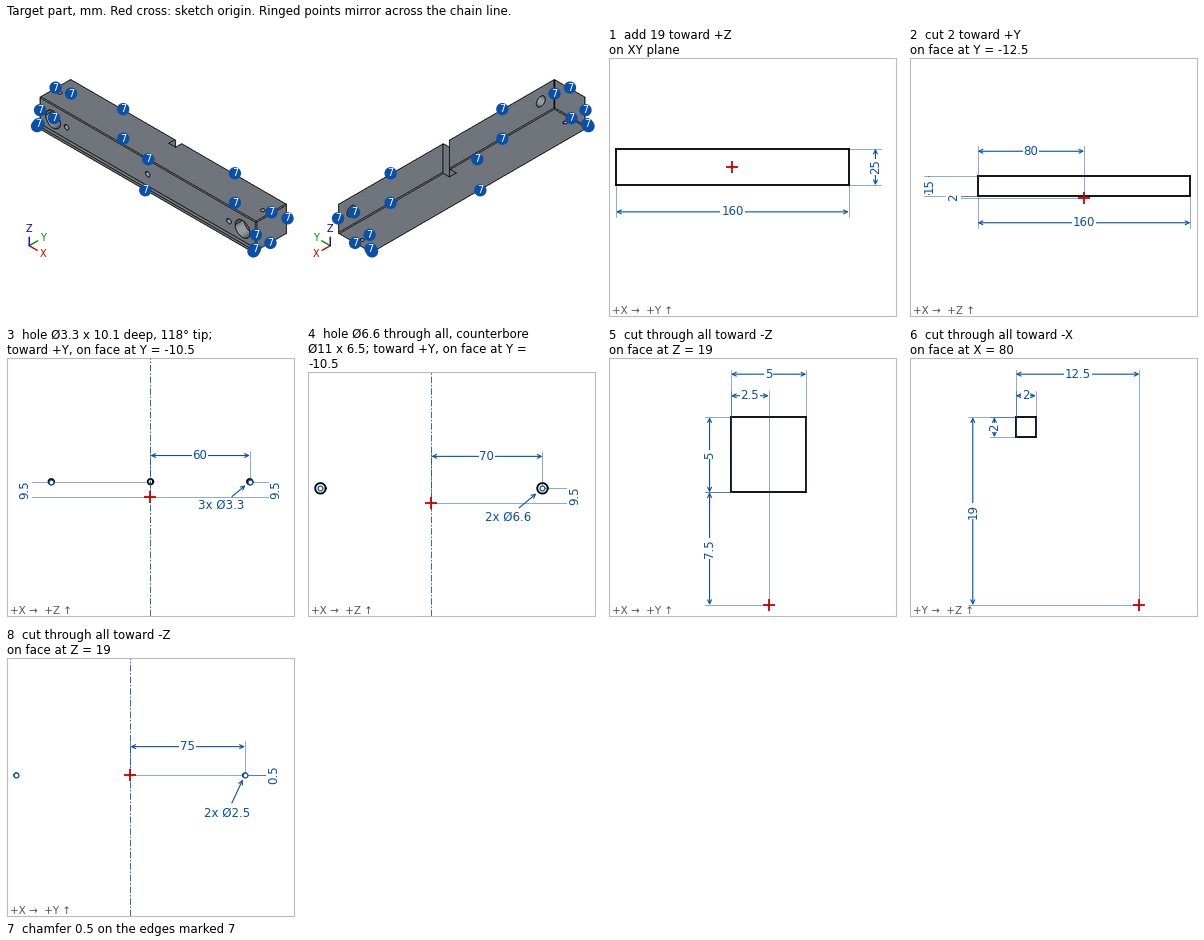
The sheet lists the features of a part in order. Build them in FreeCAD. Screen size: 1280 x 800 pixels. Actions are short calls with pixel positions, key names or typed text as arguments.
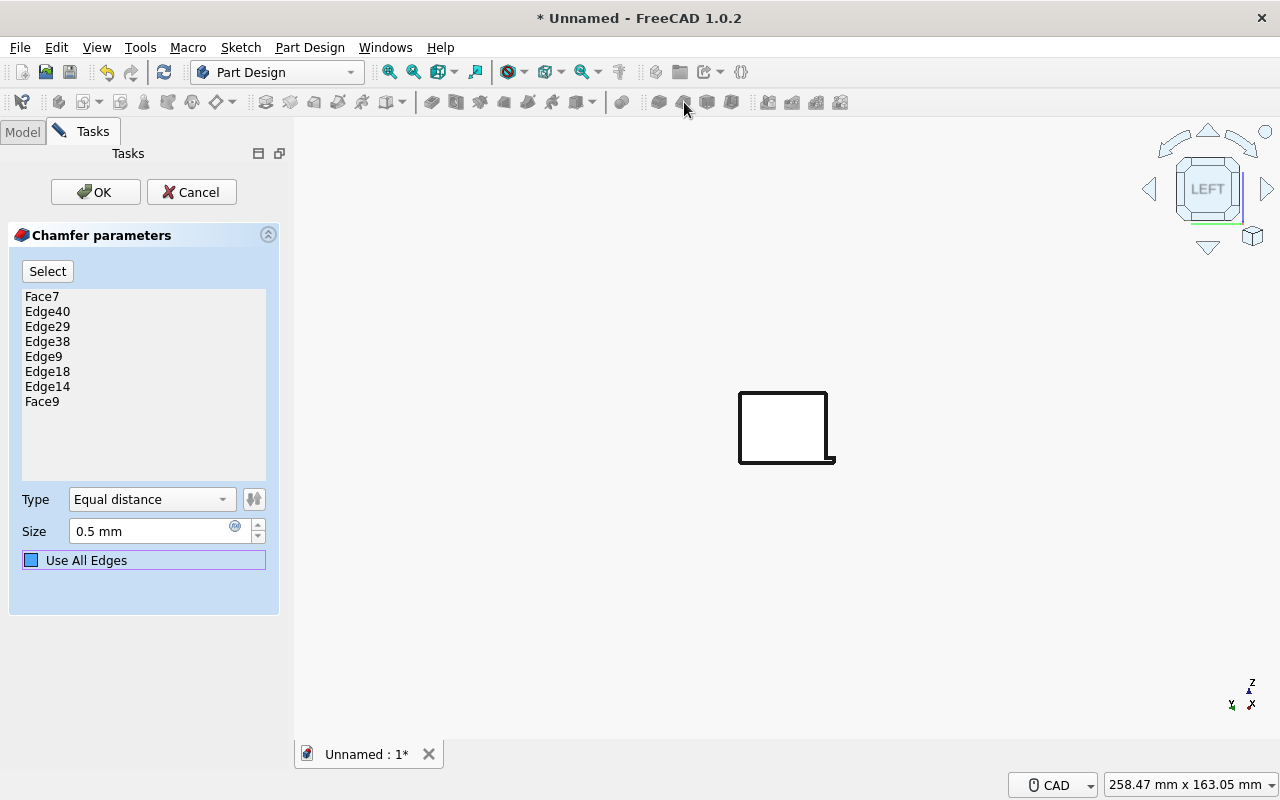
click(96, 192)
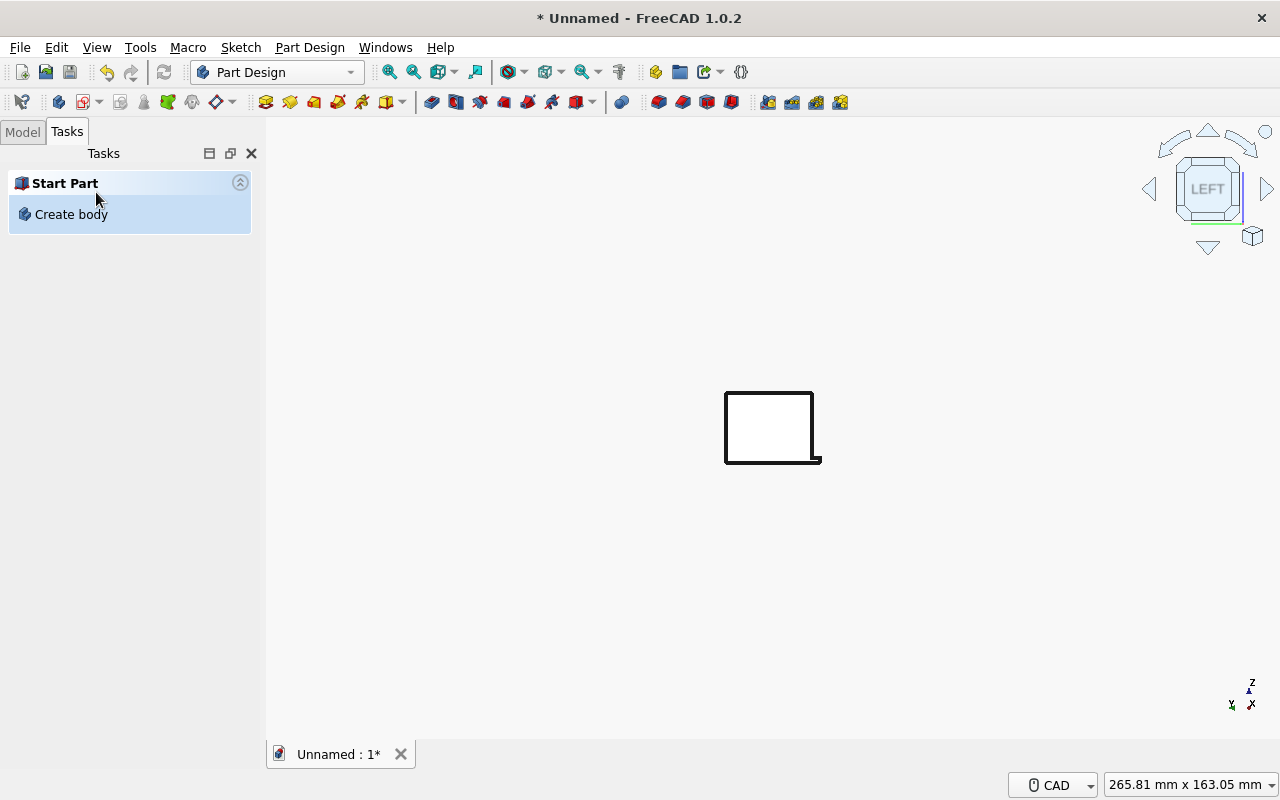
click(390, 72)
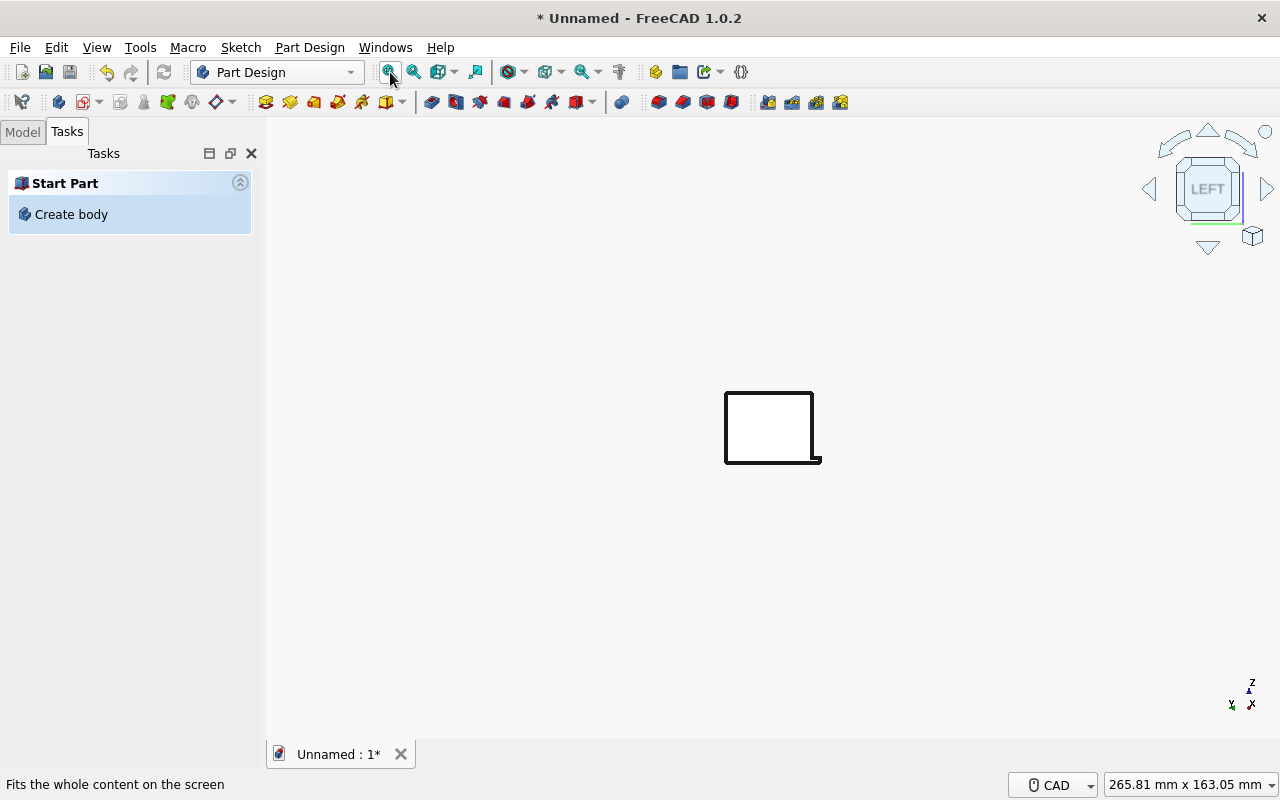
key(0)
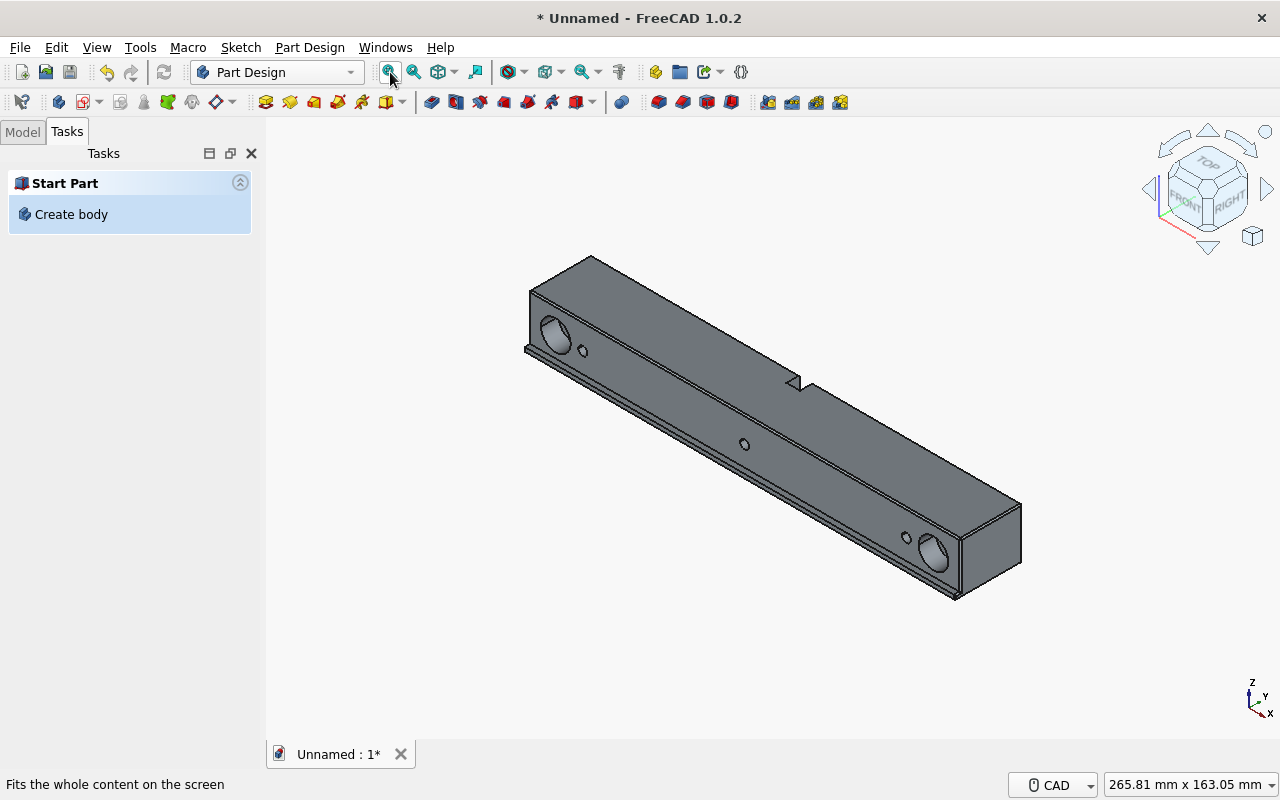
click(960, 502)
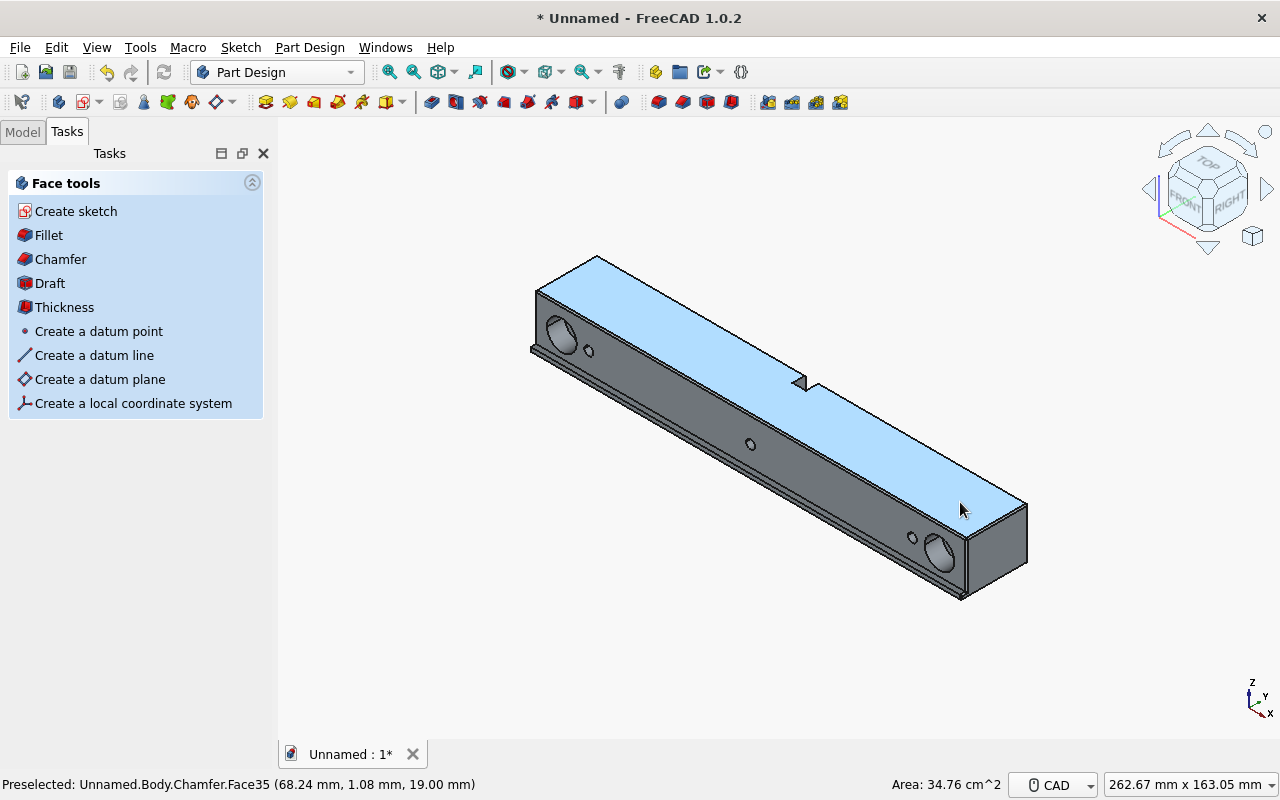
click(84, 102)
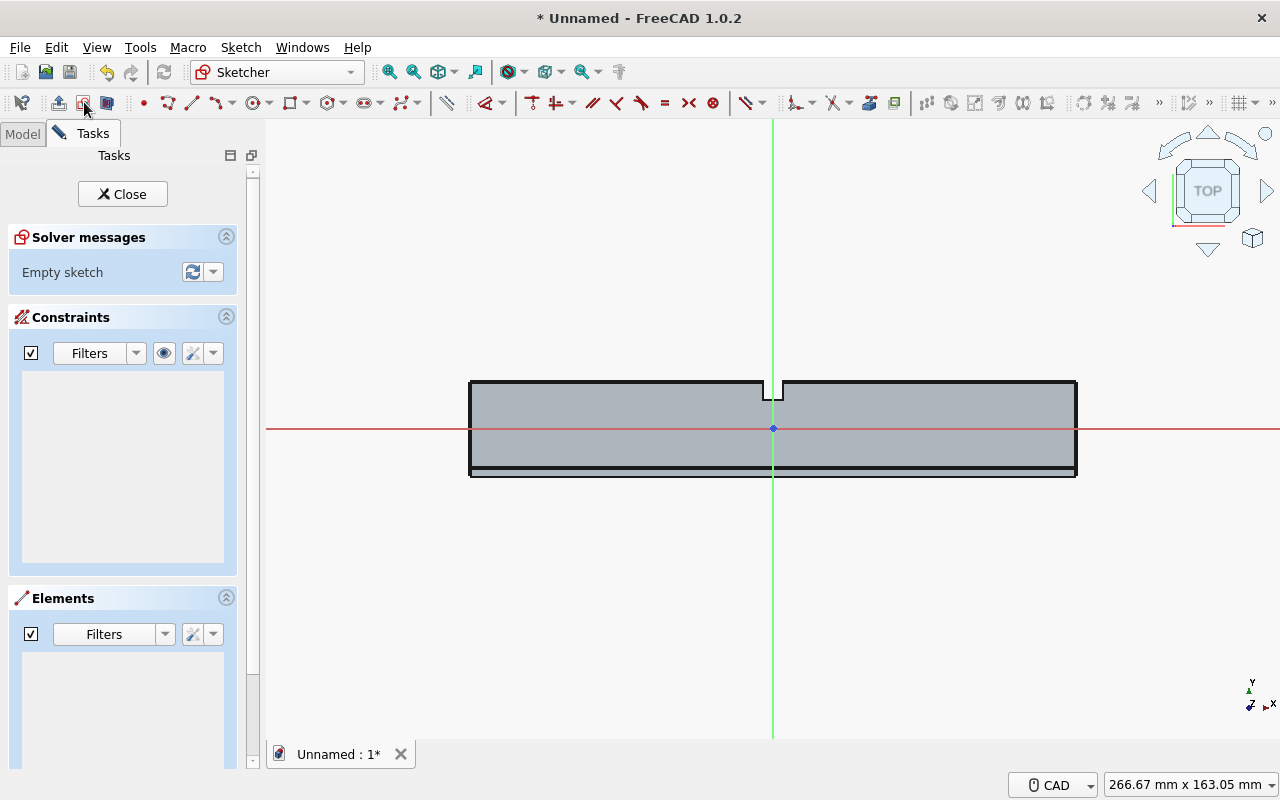
click(254, 104)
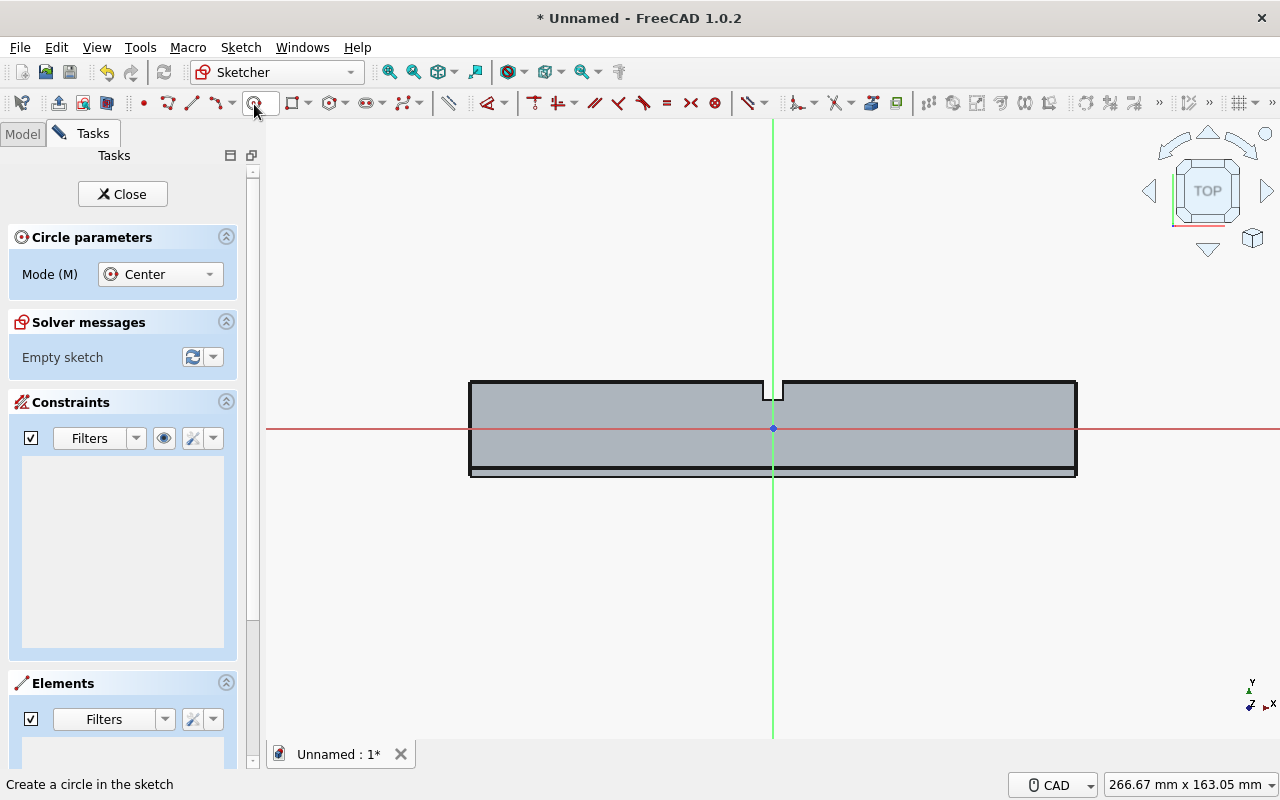
scroll(1058, 431, up, 11)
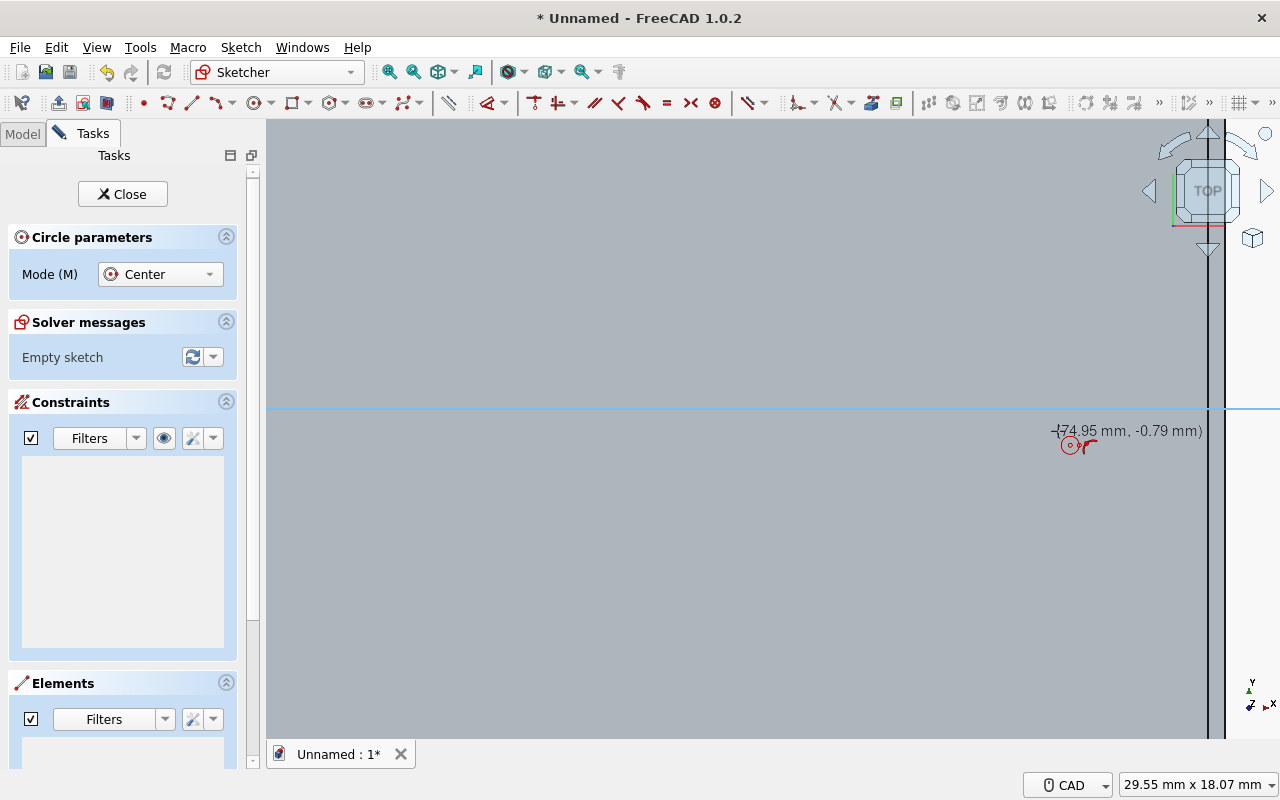
click(1053, 426)
click(1084, 456)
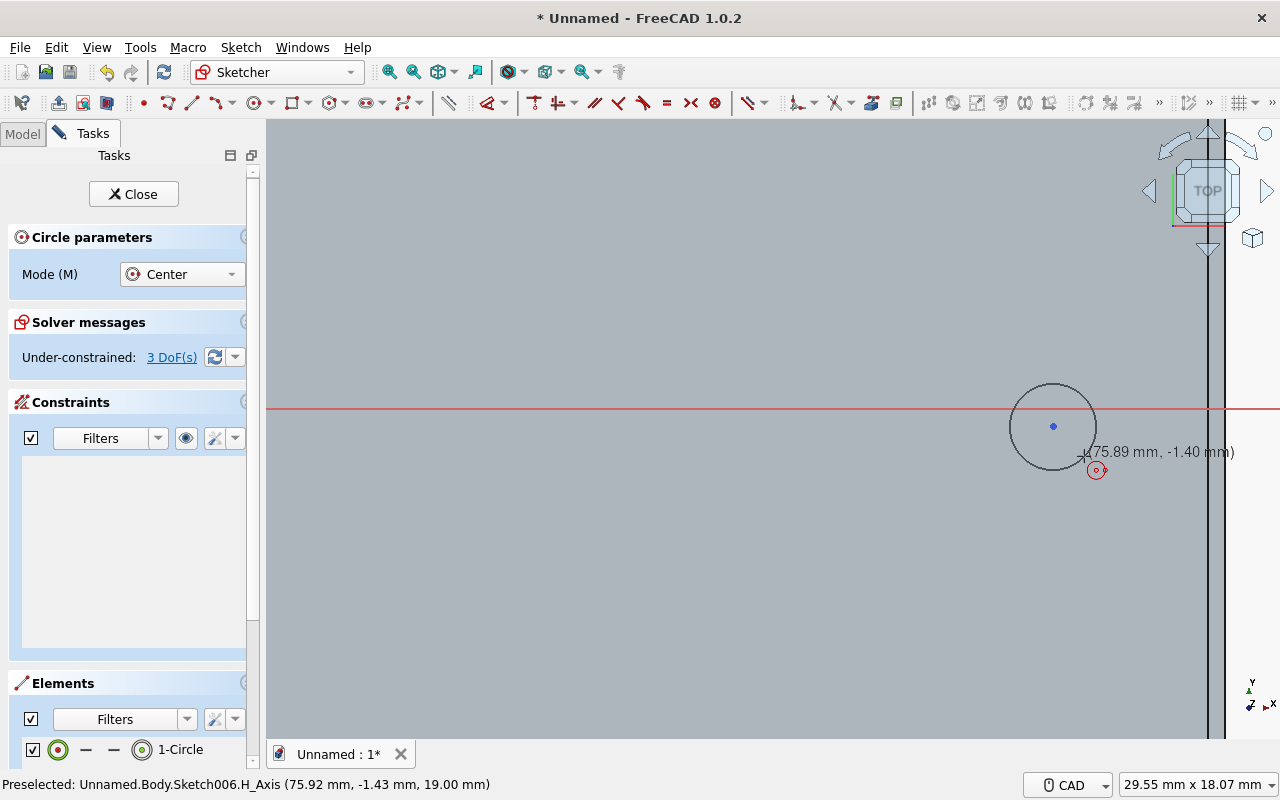
scroll(982, 429, down, 11)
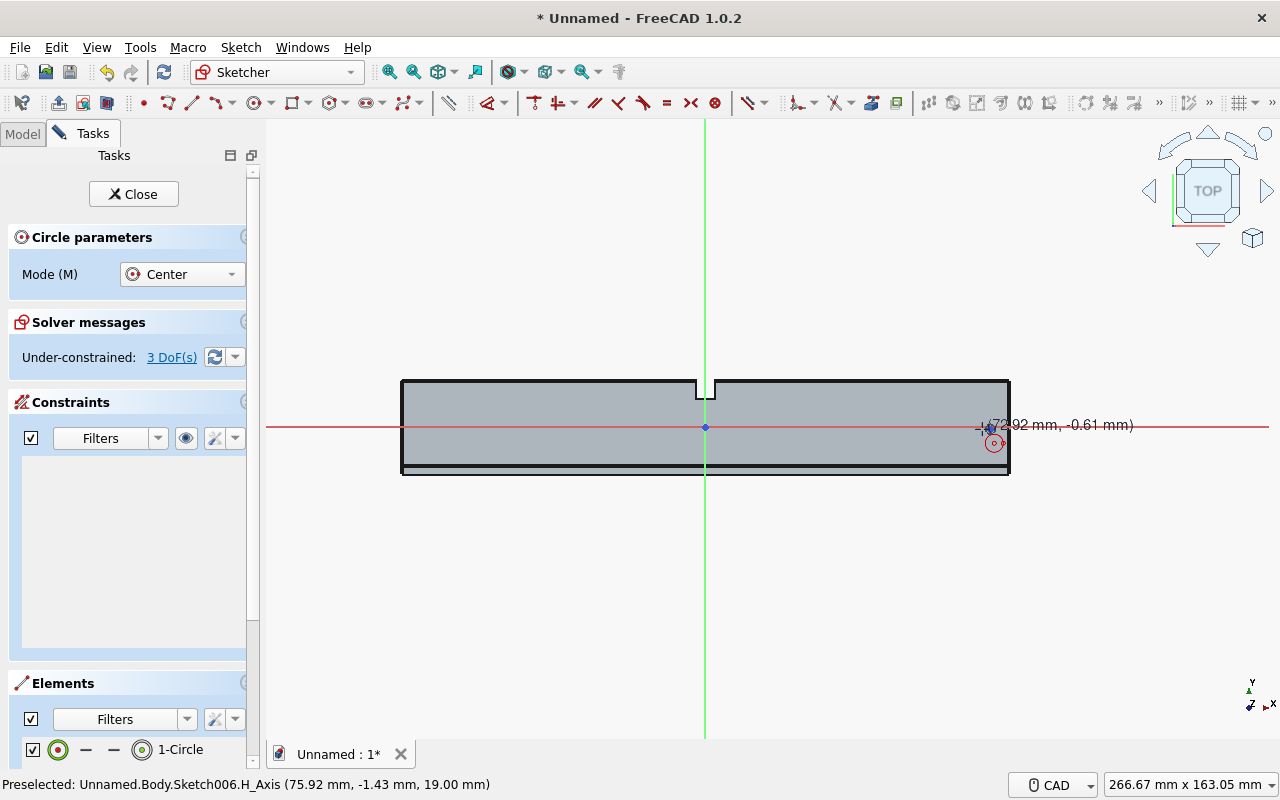
scroll(420, 429, up, 11)